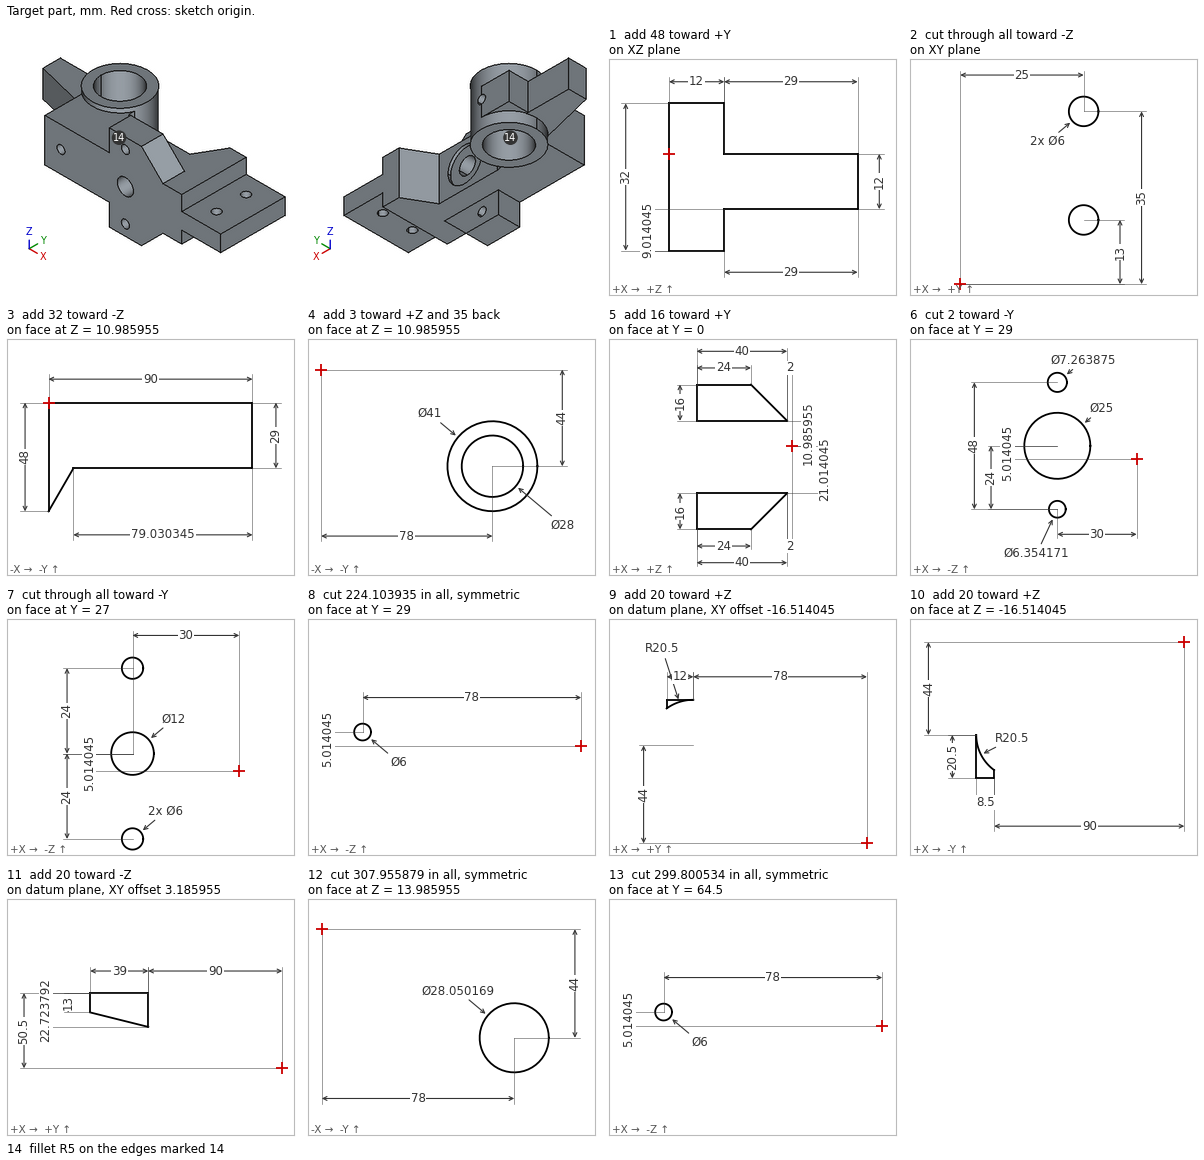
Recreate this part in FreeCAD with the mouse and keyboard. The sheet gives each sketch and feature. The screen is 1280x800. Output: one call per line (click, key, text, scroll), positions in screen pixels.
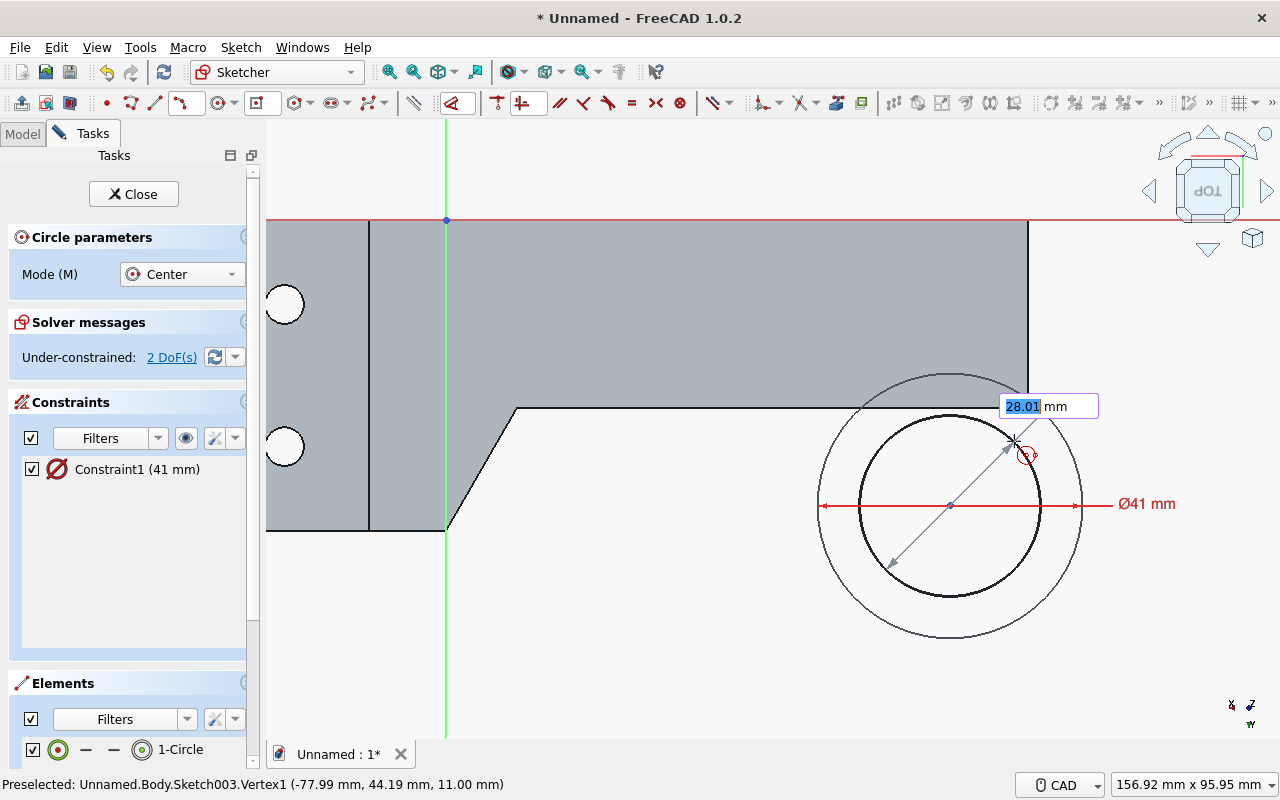
text(28)
key(Return)
key(Escape)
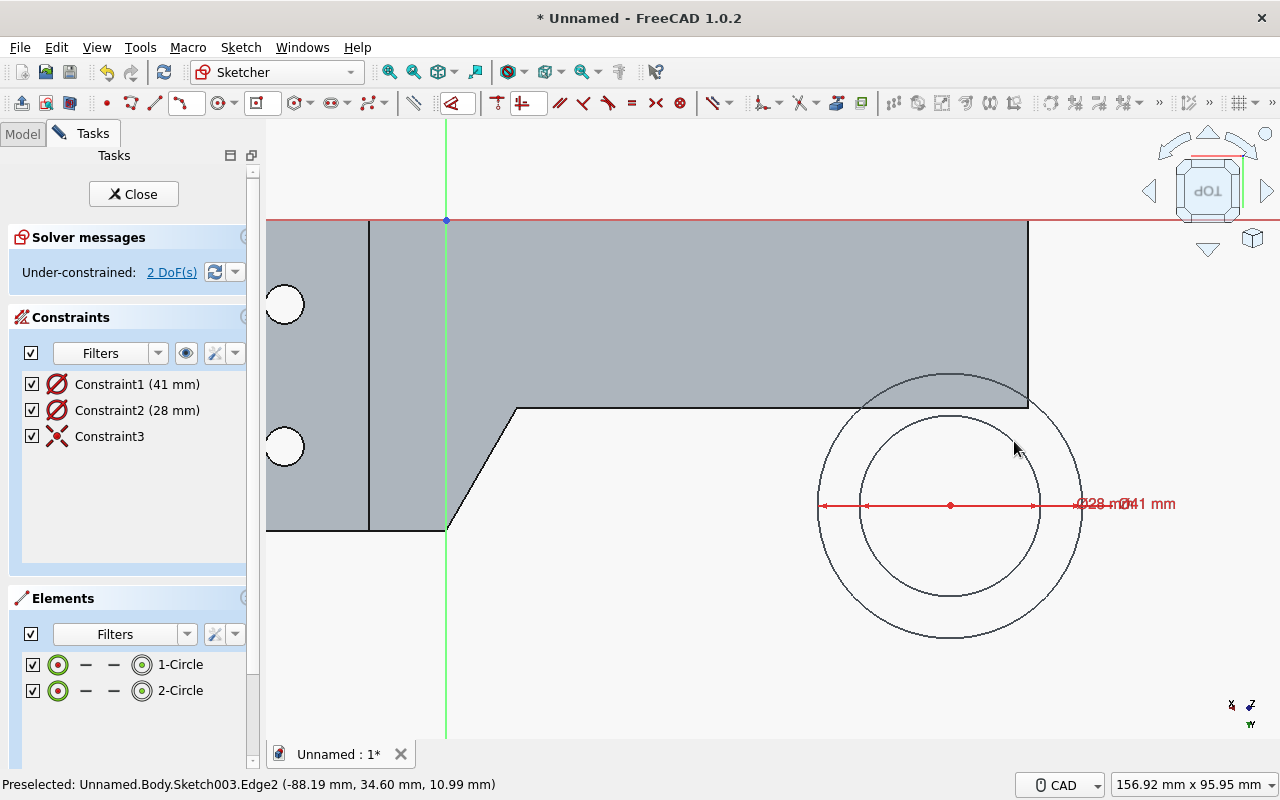
click(950, 506)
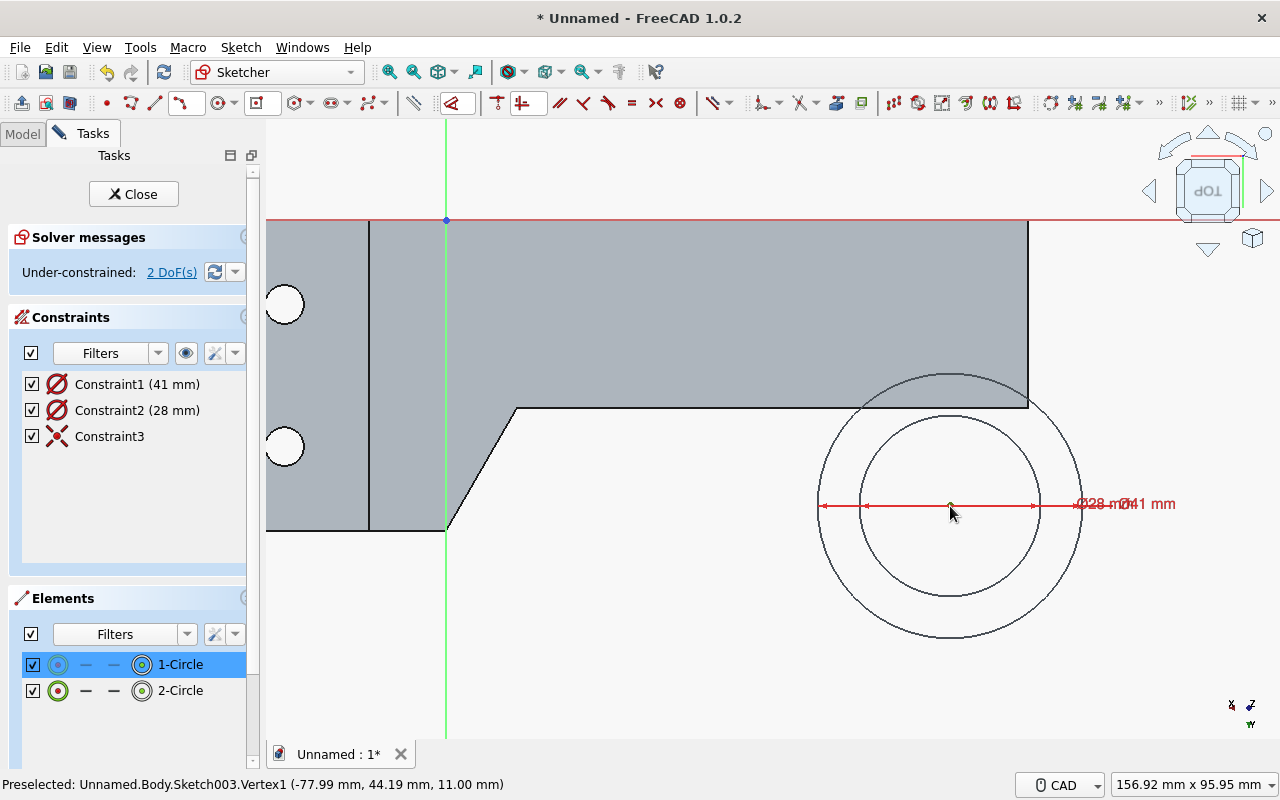
key(l)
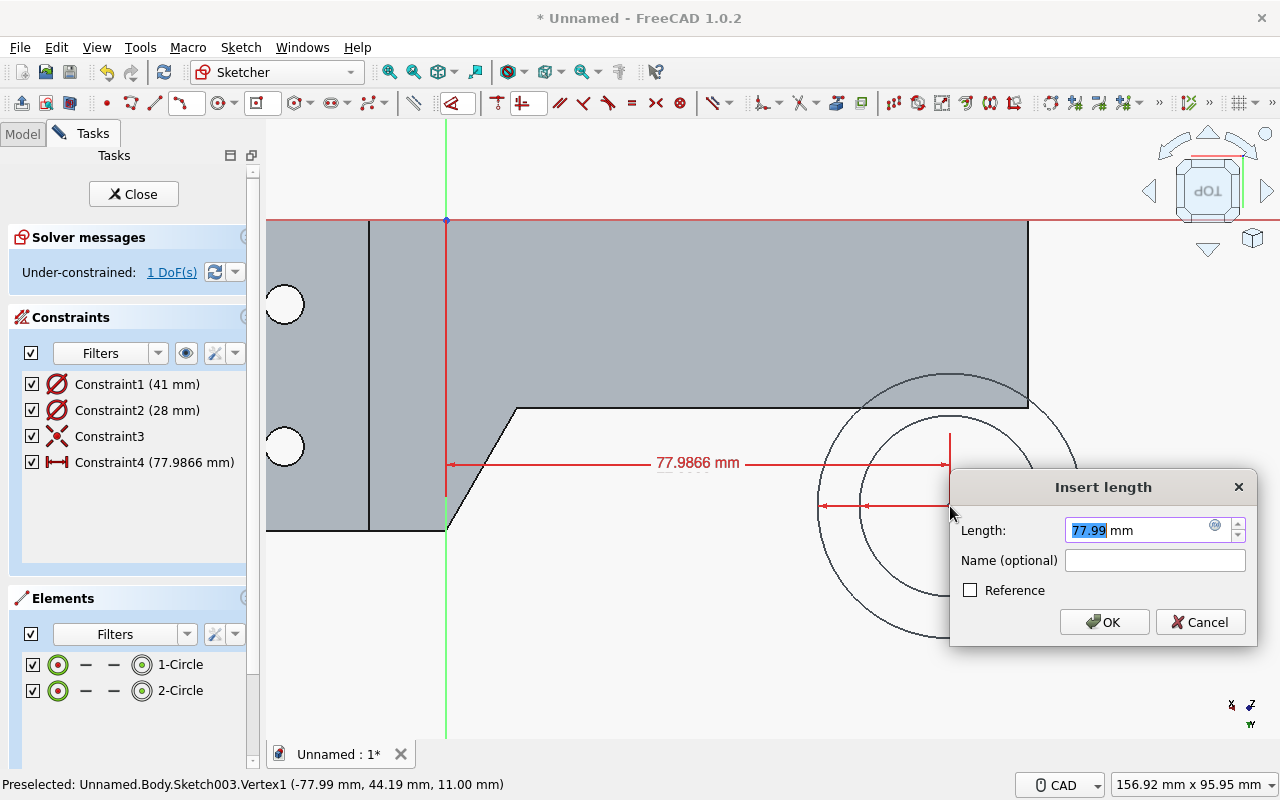
text(78)
key(Return)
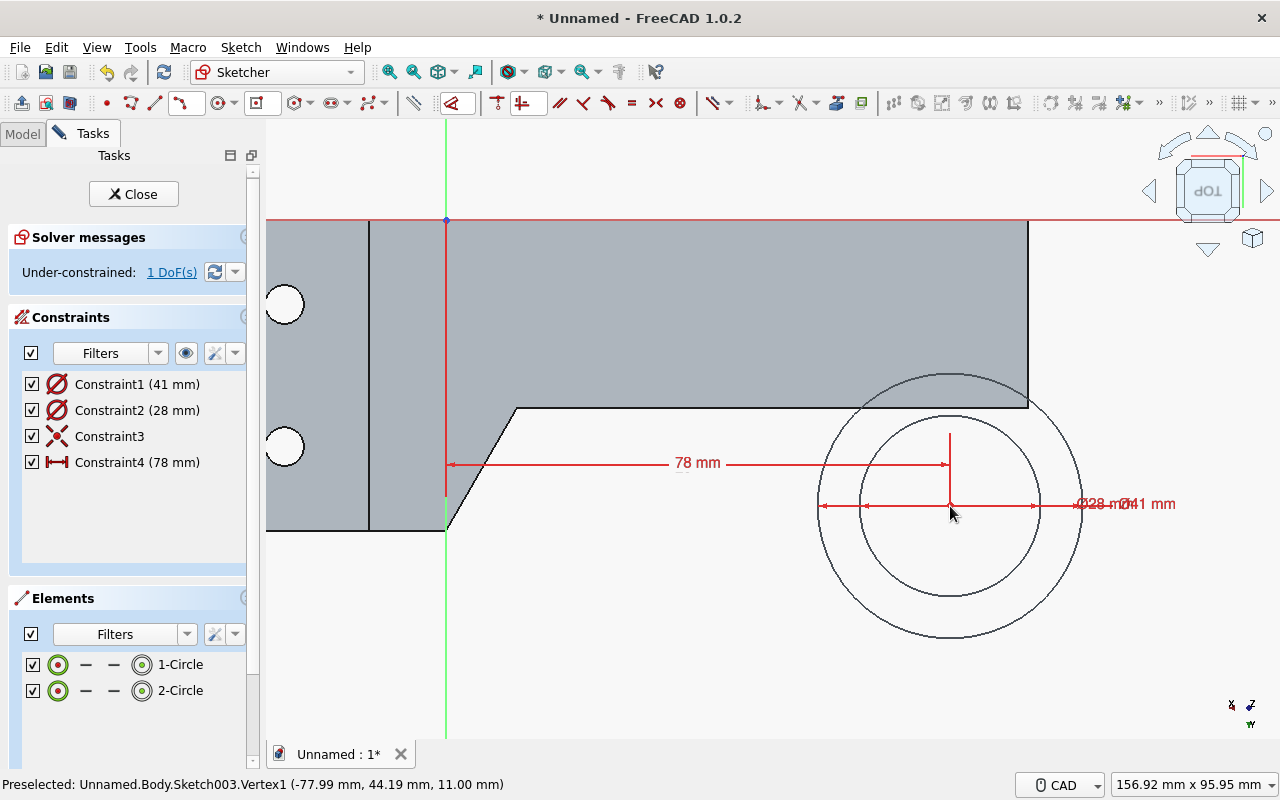
click(950, 506)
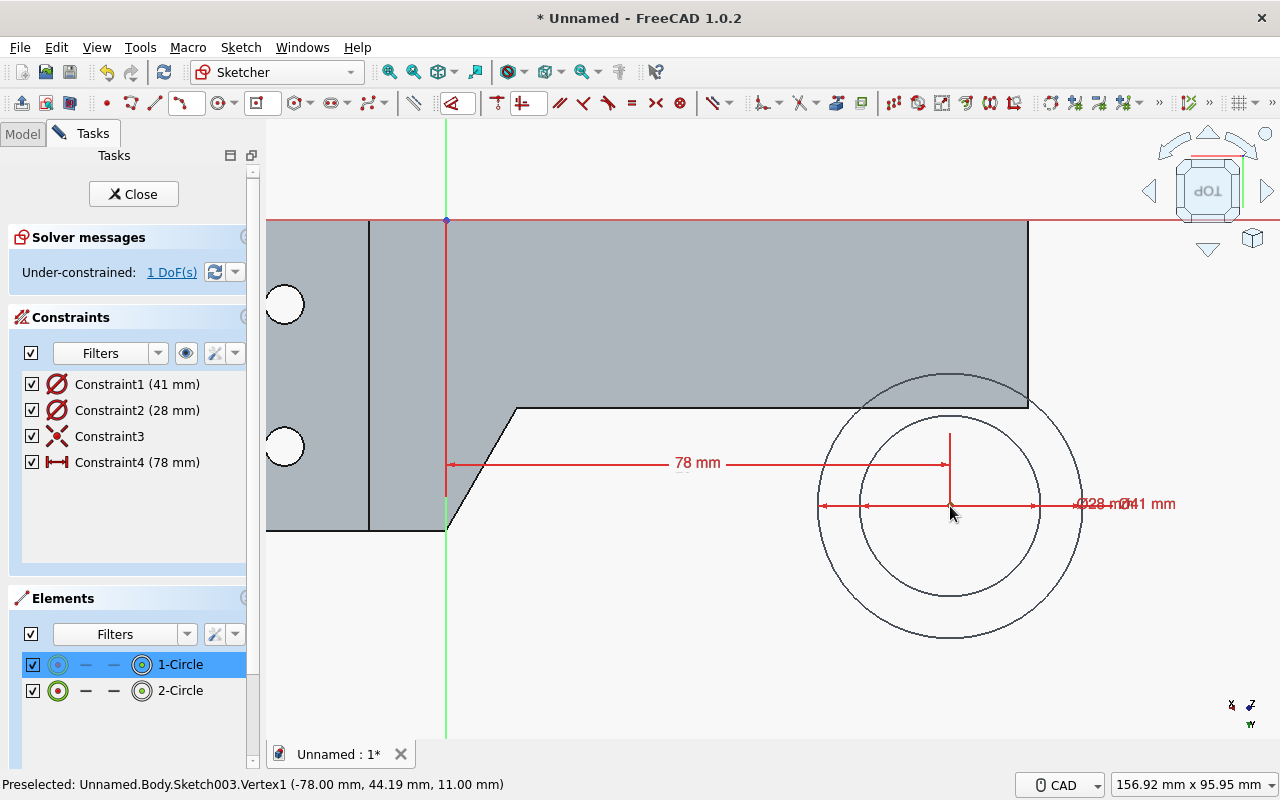
key(i)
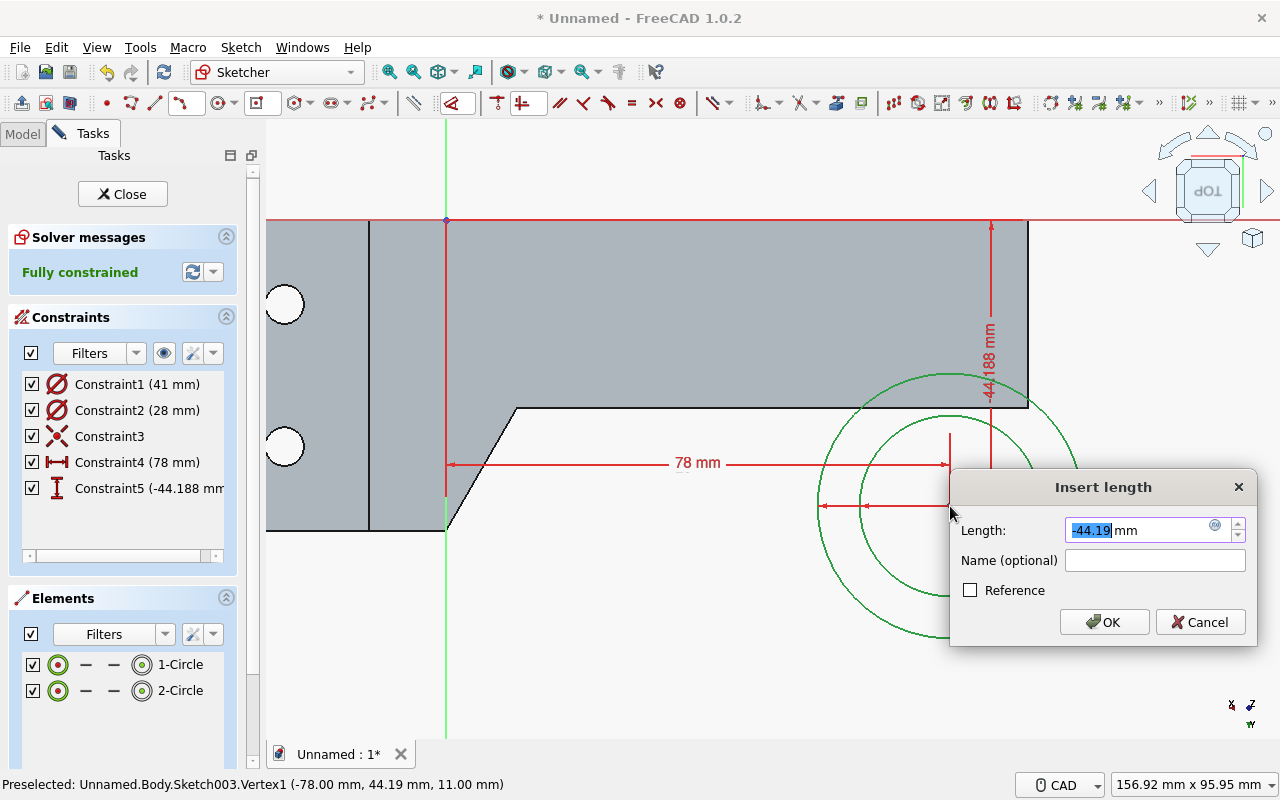
text(-44)
key(Return)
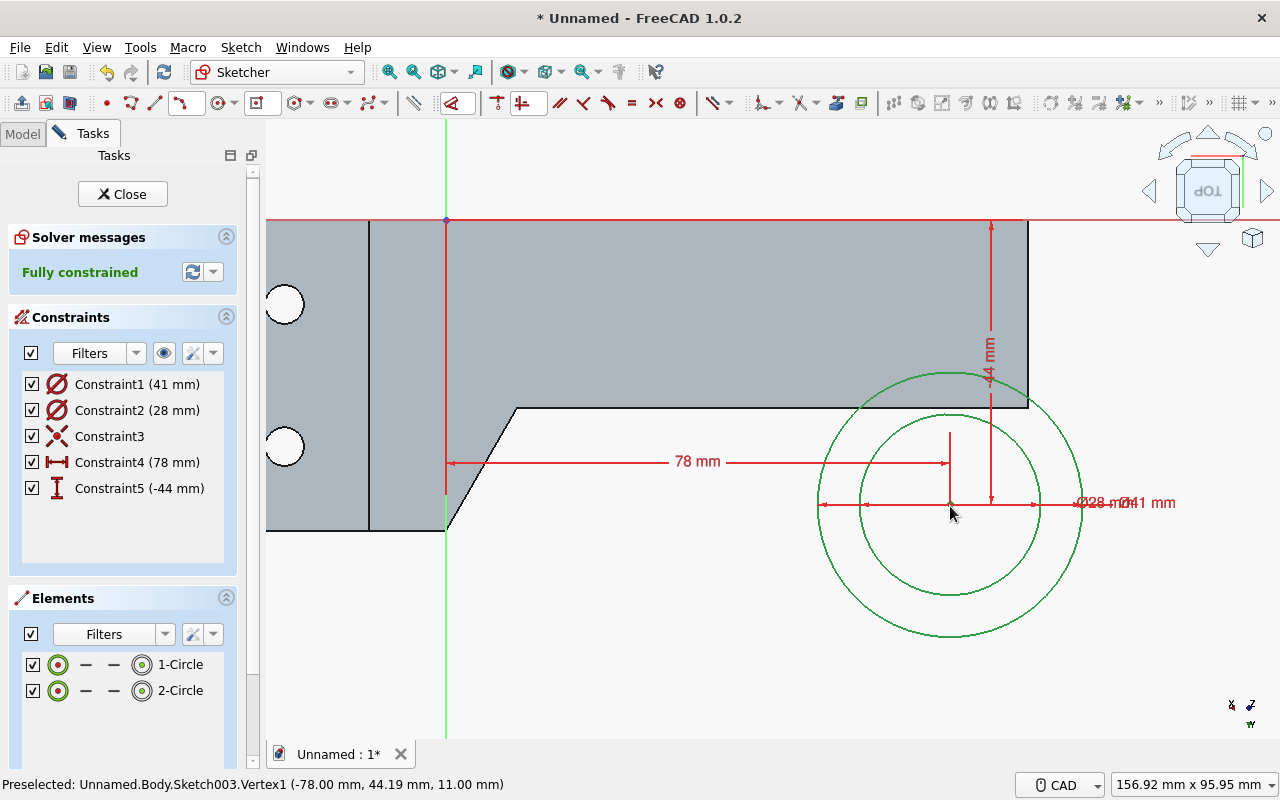
click(123, 194)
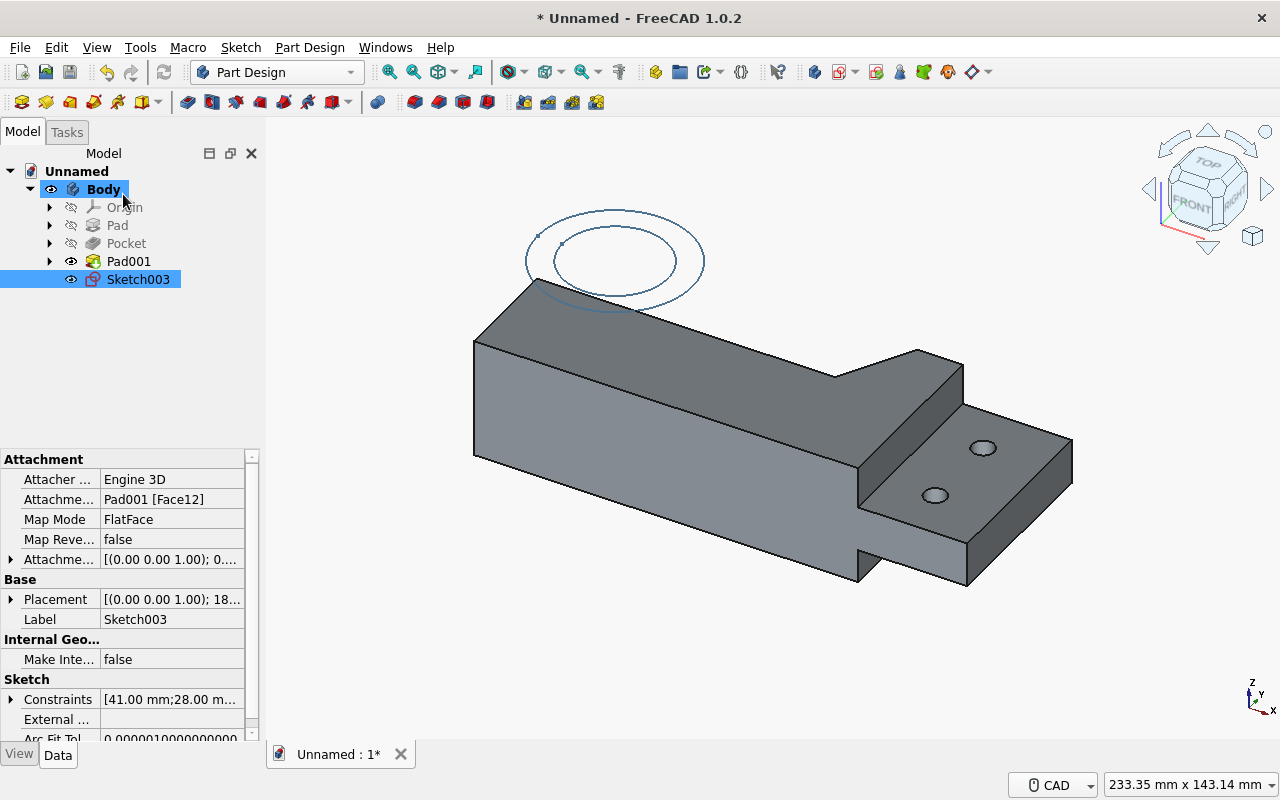
click(22, 102)